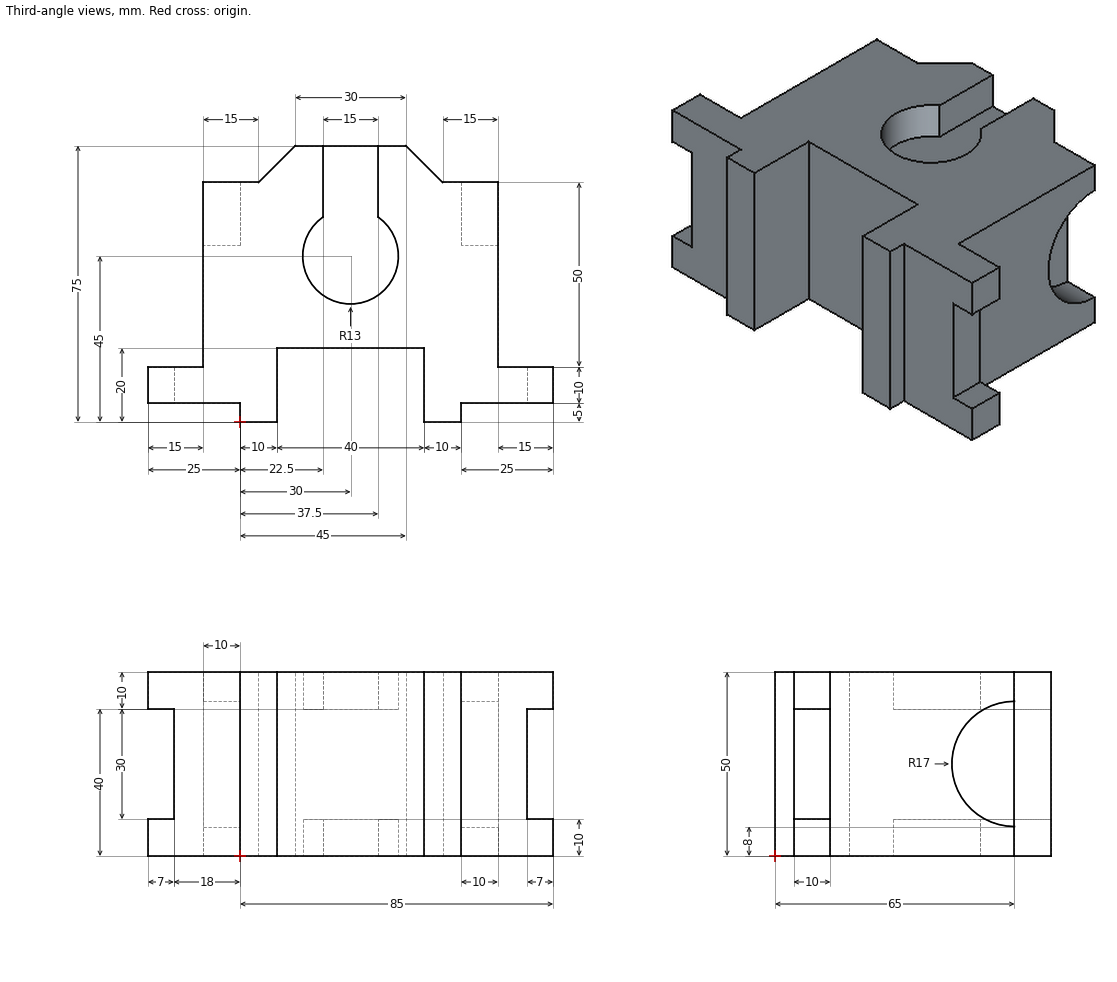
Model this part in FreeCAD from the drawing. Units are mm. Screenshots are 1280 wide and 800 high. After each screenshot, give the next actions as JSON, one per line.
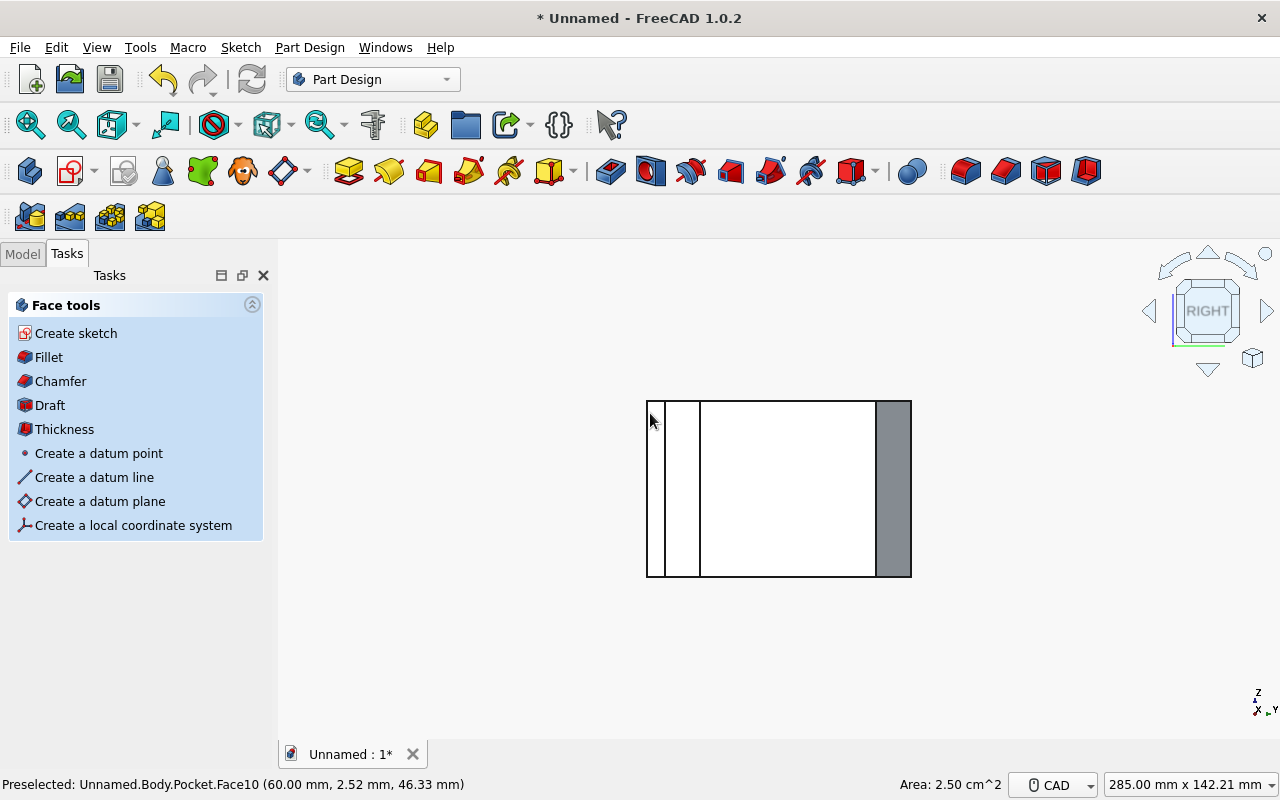
{"action": "left_click", "coordinate": [70, 172]}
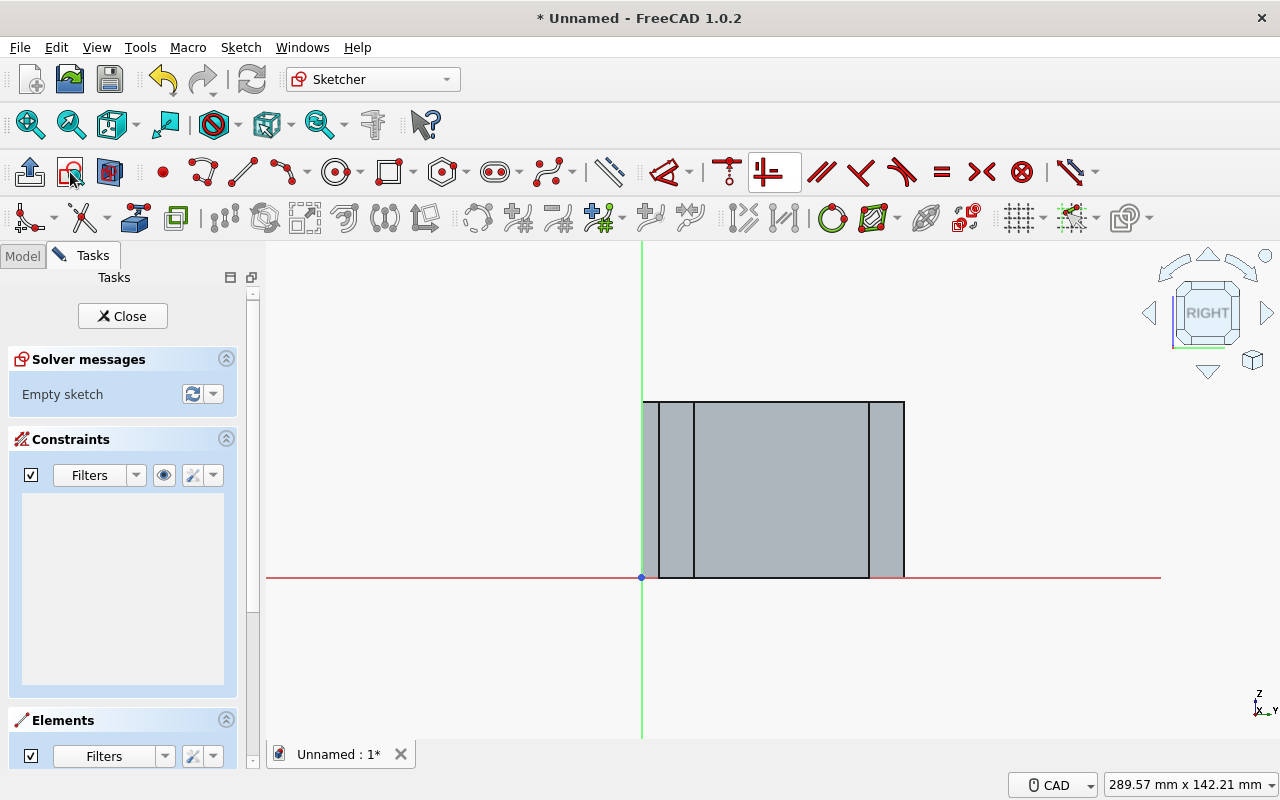
{"action": "left_click", "coordinate": [110, 172]}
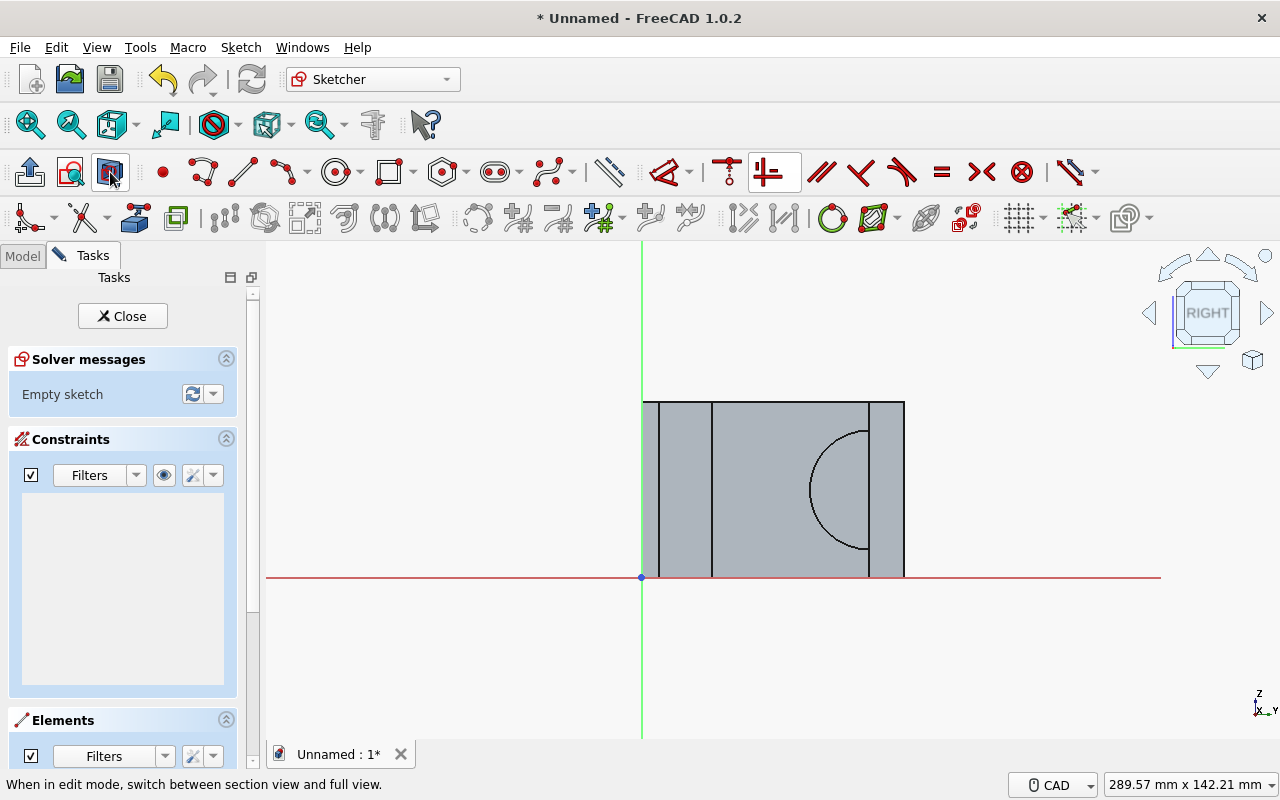
{"action": "scroll", "coordinate": [797, 515], "scroll_direction": "up", "scroll_amount": 4}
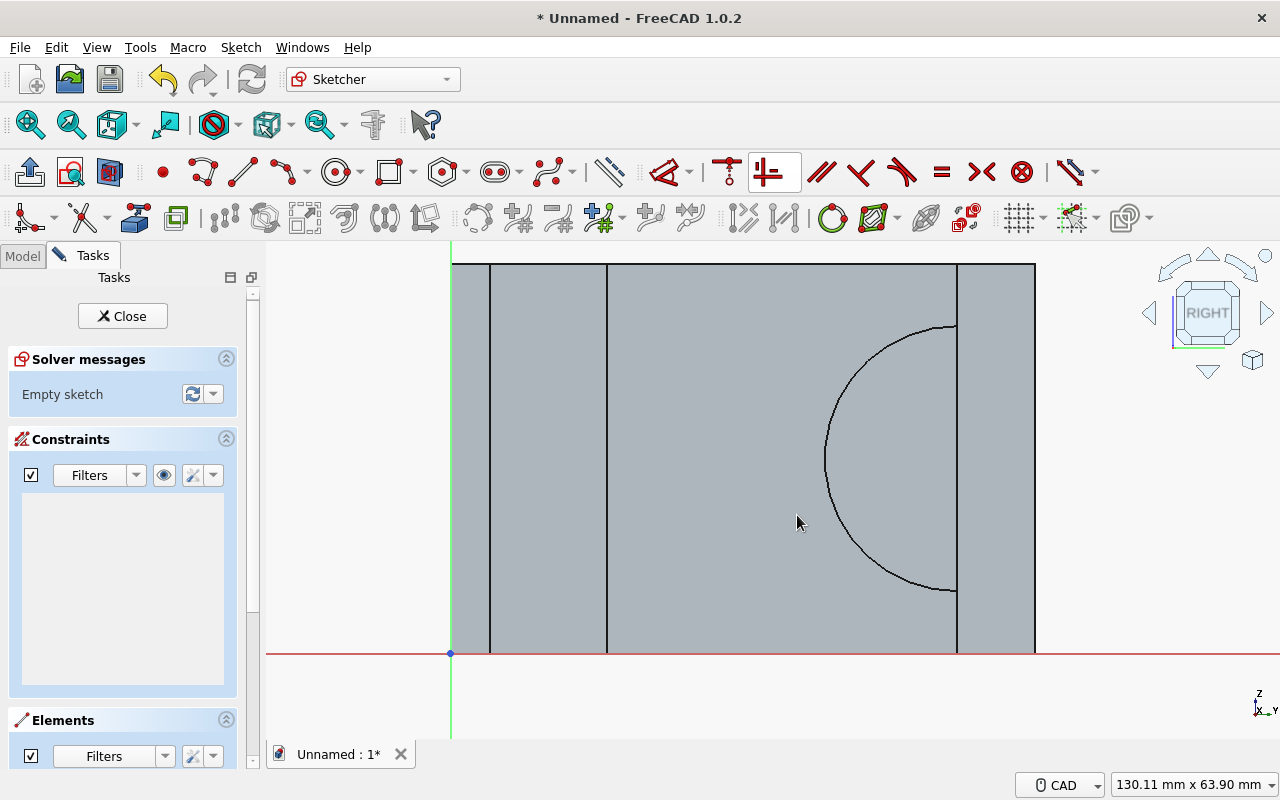
{"action": "left_click", "coordinate": [244, 172]}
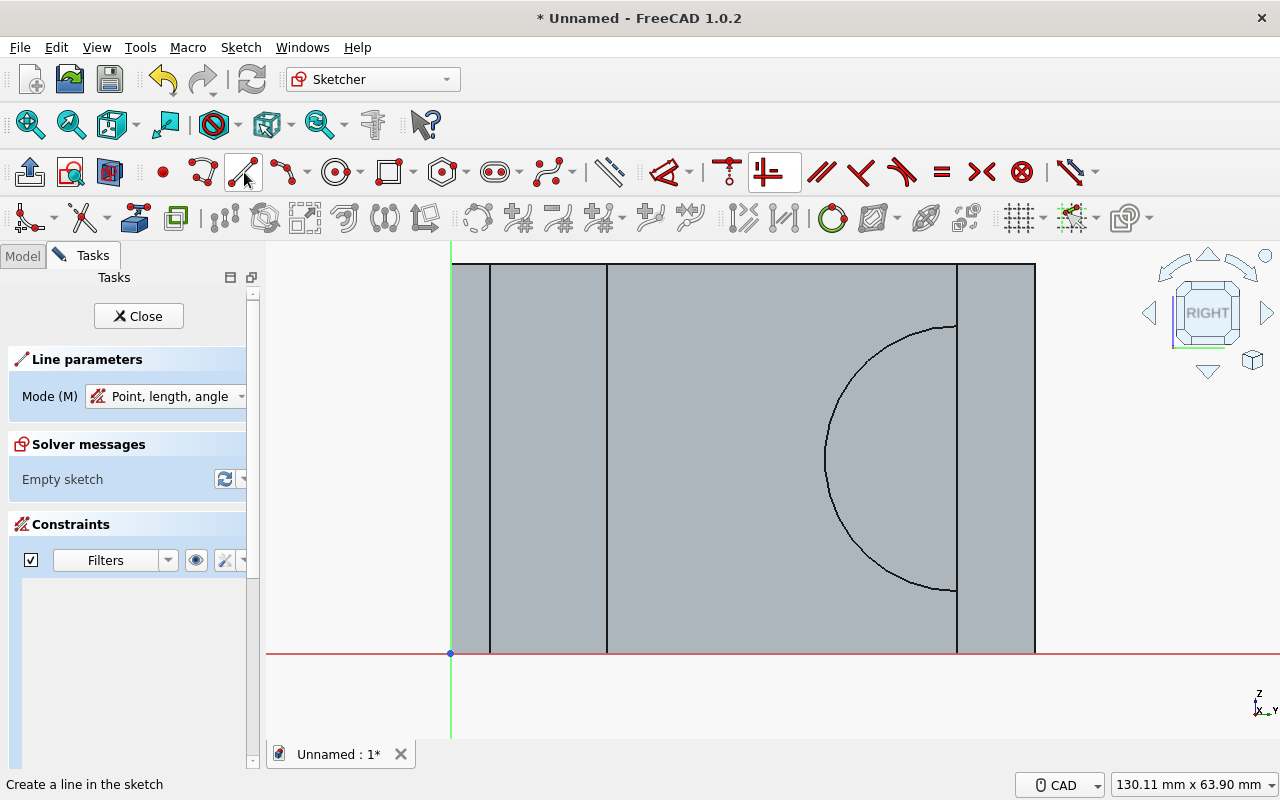
{"action": "left_click", "coordinate": [957, 591]}
{"action": "left_click", "coordinate": [957, 326]}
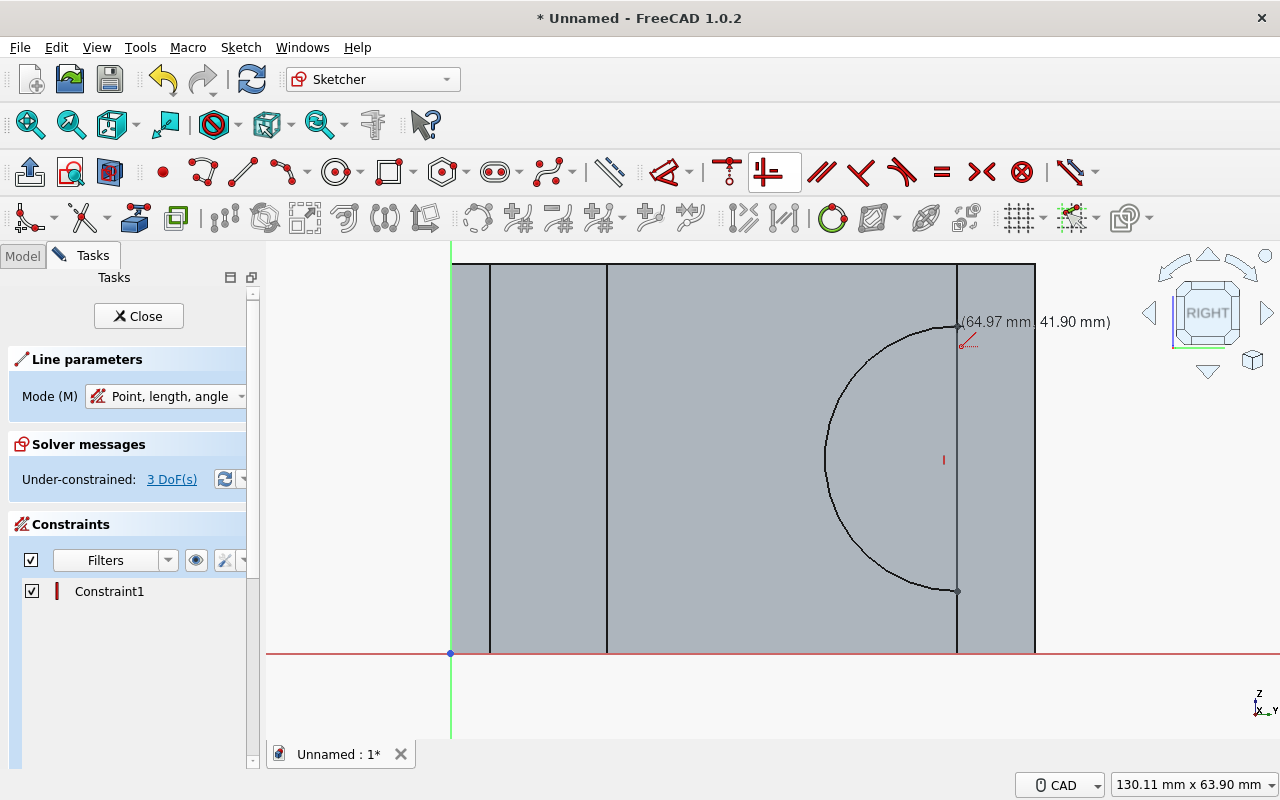
{"action": "left_click", "coordinate": [284, 172]}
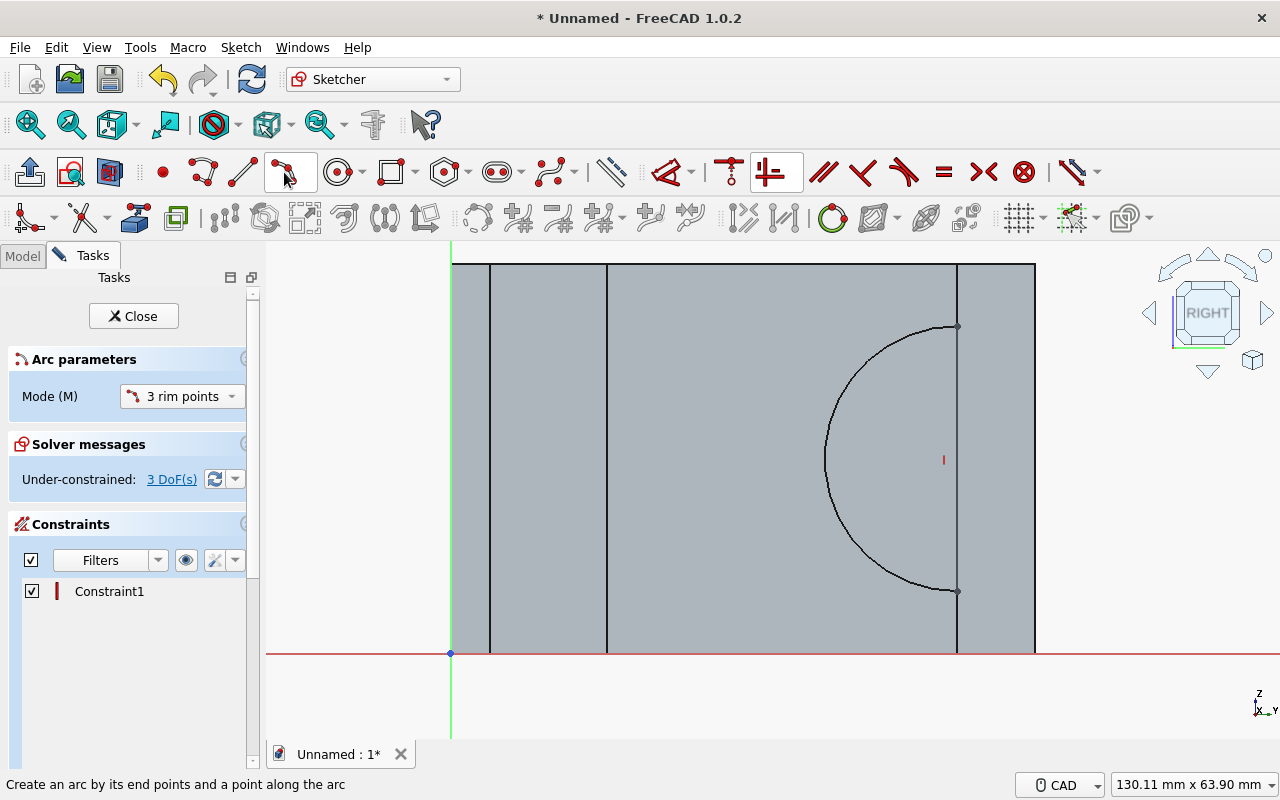
{"action": "left_click", "coordinate": [957, 327]}
{"action": "left_click", "coordinate": [957, 592]}
{"action": "left_click", "coordinate": [825, 459]}
{"action": "key", "text": "Escape"}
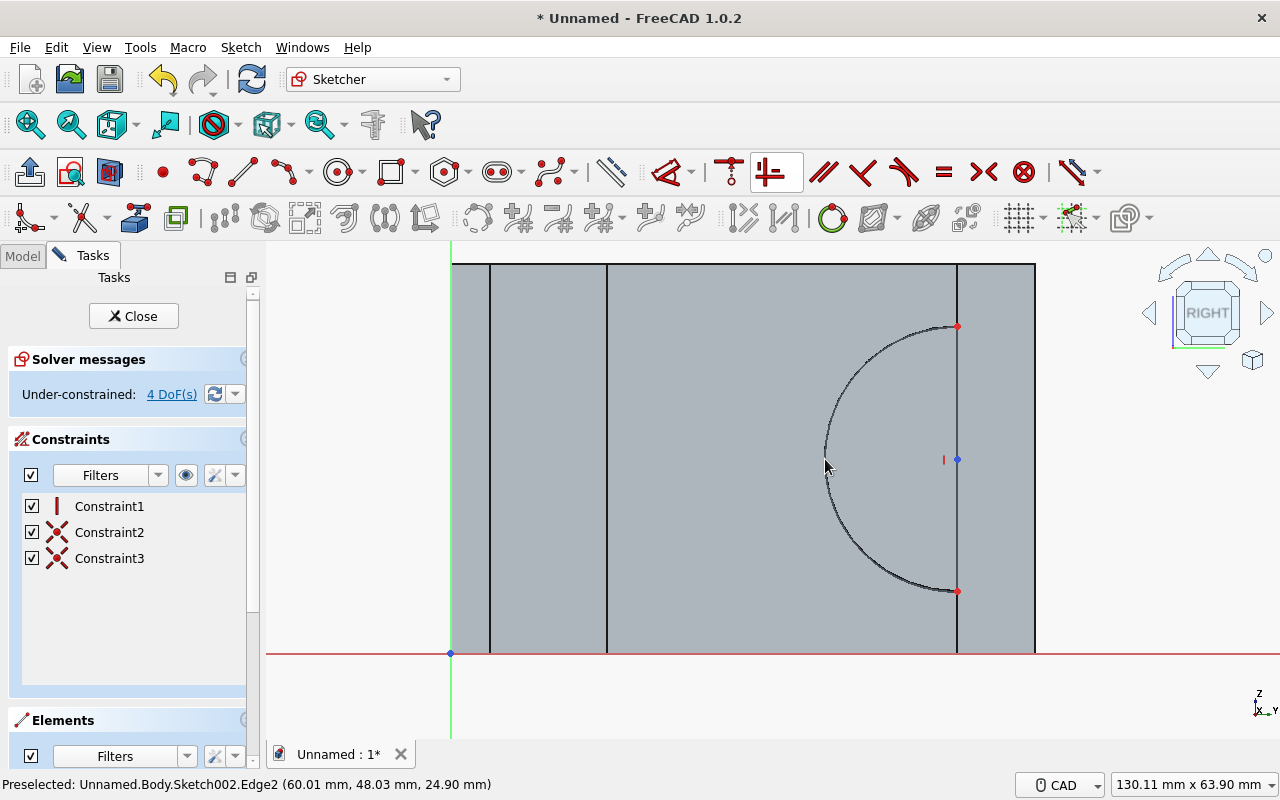
{"action": "left_click", "coordinate": [666, 172]}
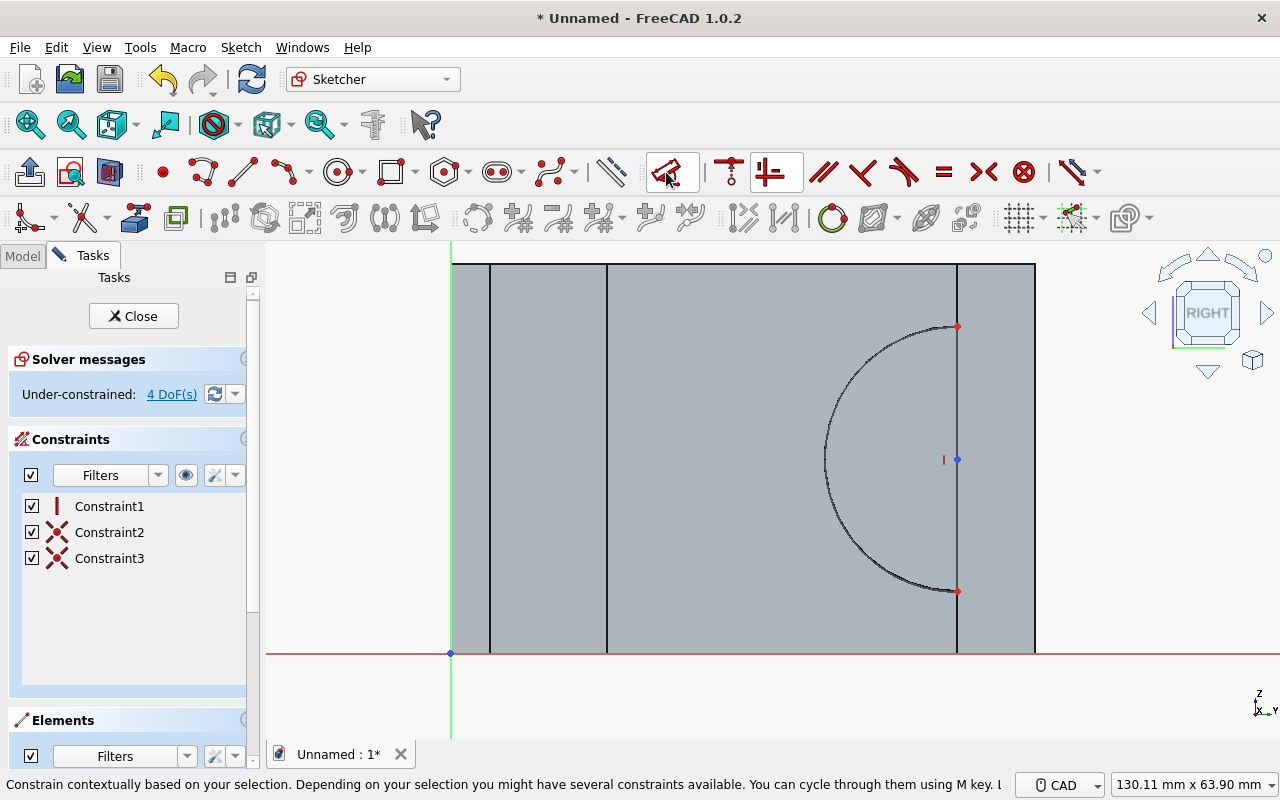
{"action": "left_click", "coordinate": [850, 382]}
{"action": "left_click", "coordinate": [824, 363]}